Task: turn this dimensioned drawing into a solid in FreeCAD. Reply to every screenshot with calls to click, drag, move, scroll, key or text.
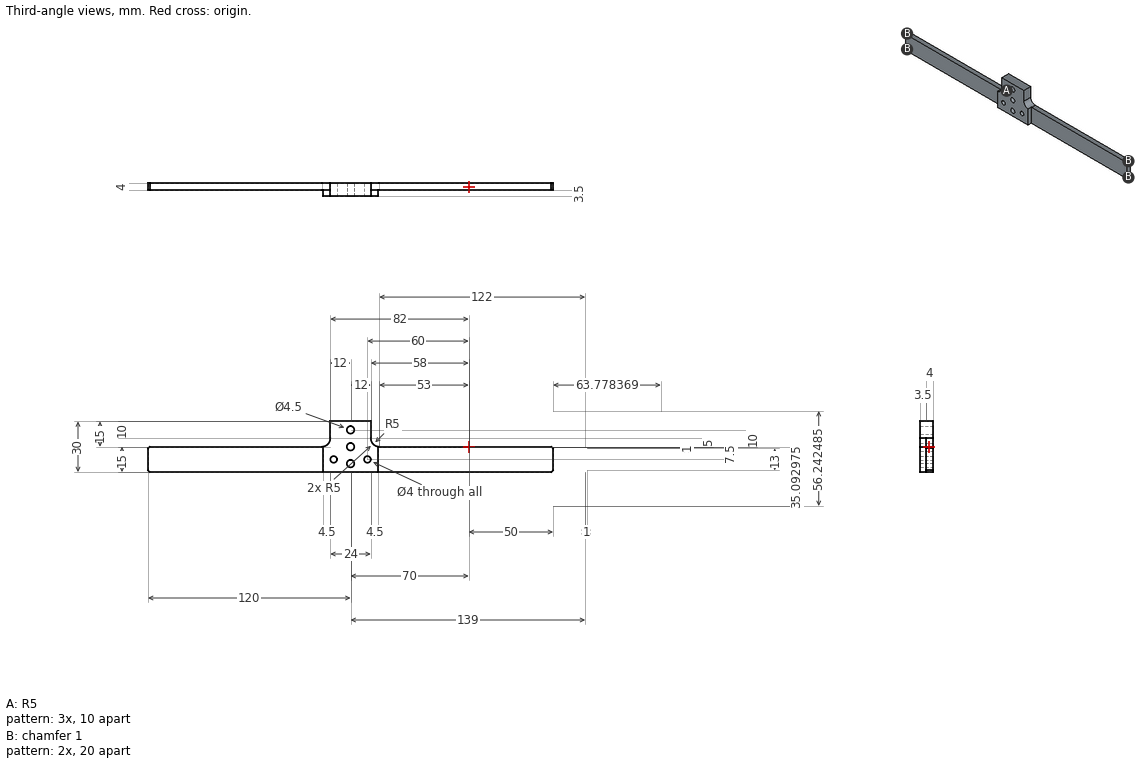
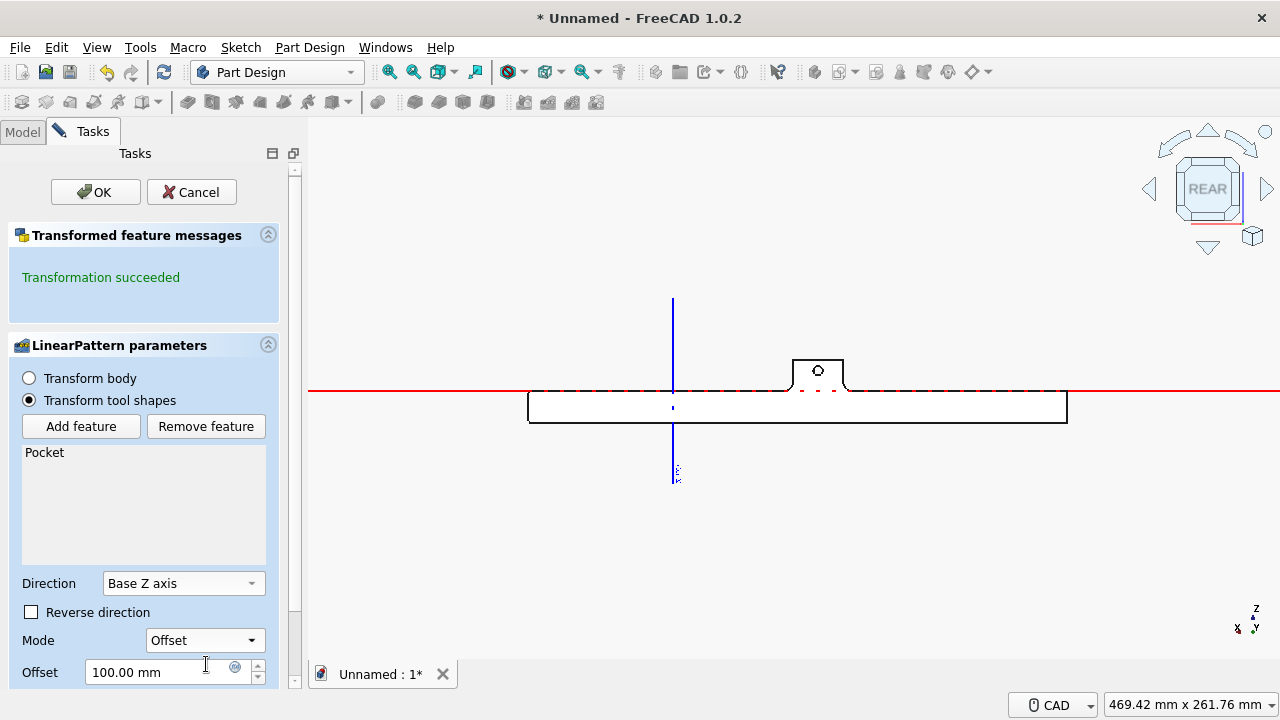
triple_click(168, 672)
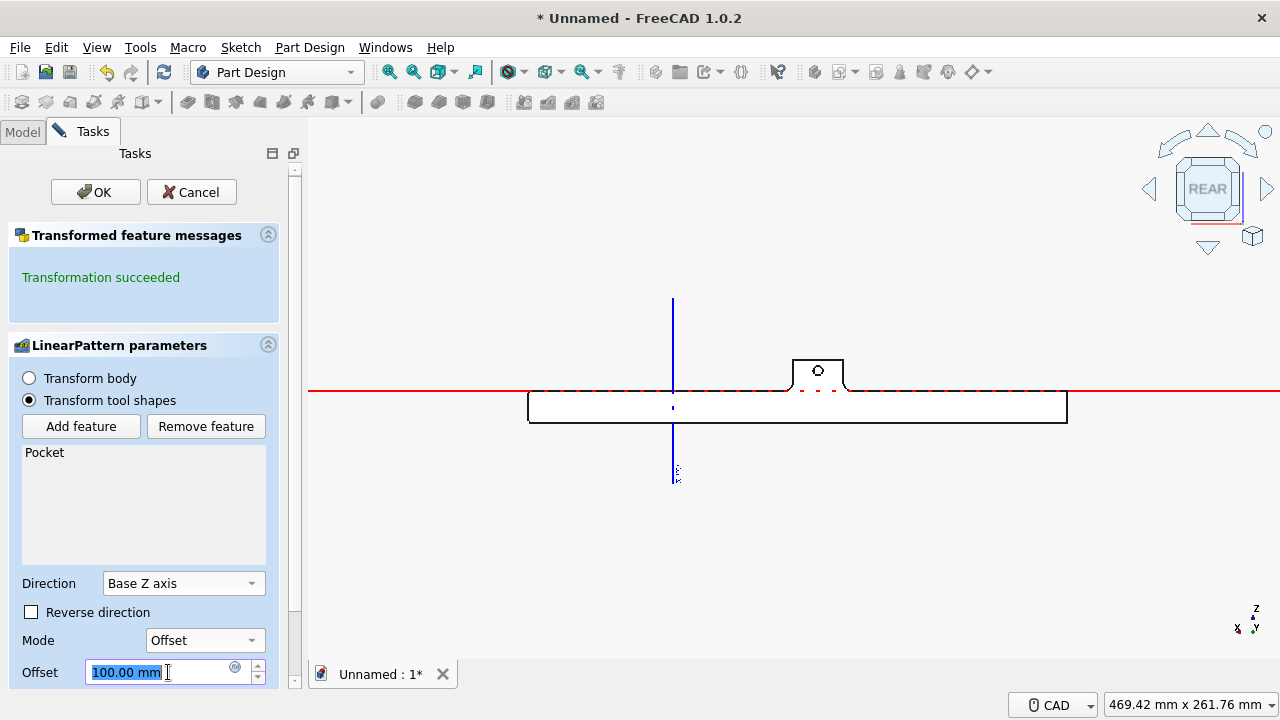
text(10)
key(Tab)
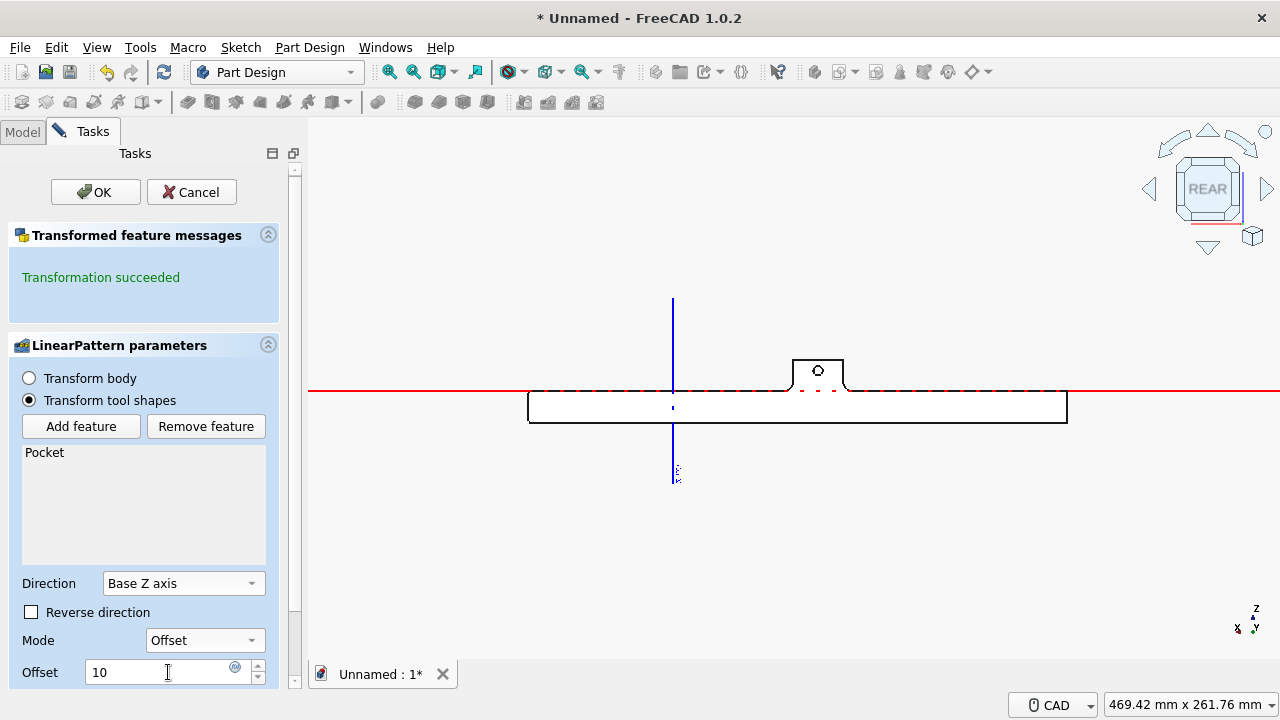
scroll(295, 426, down, 2)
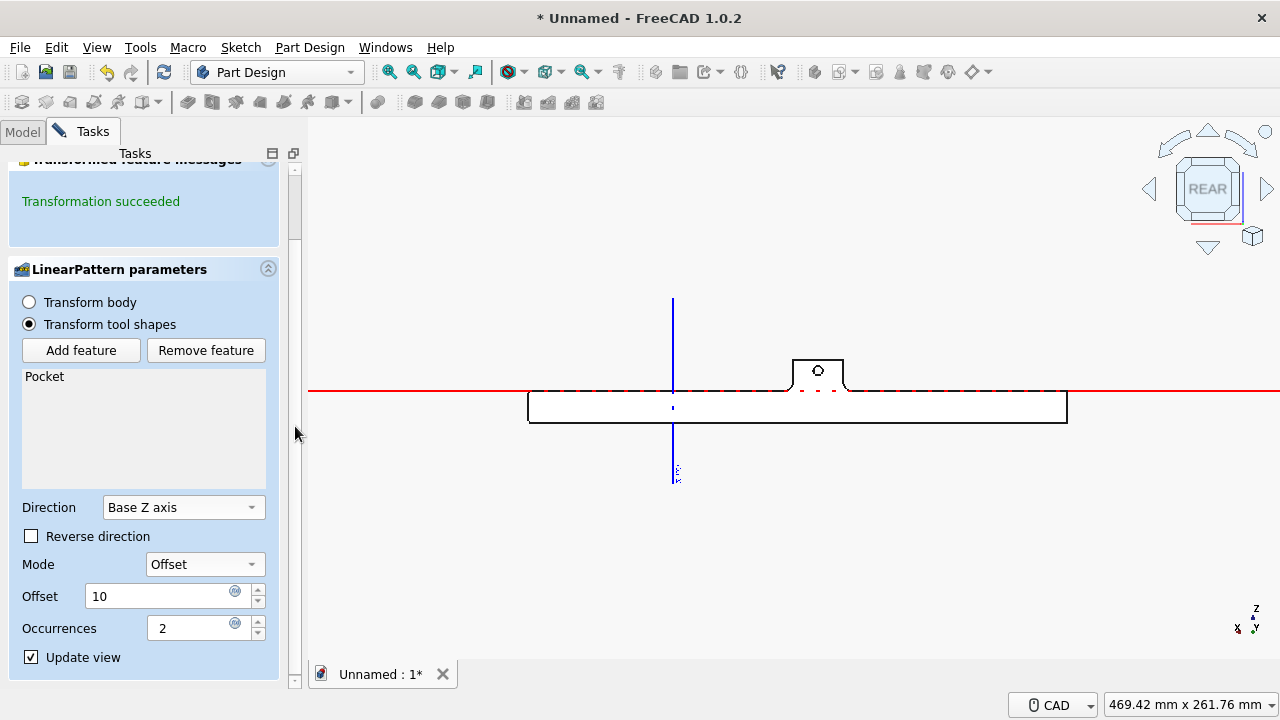
triple_click(198, 628)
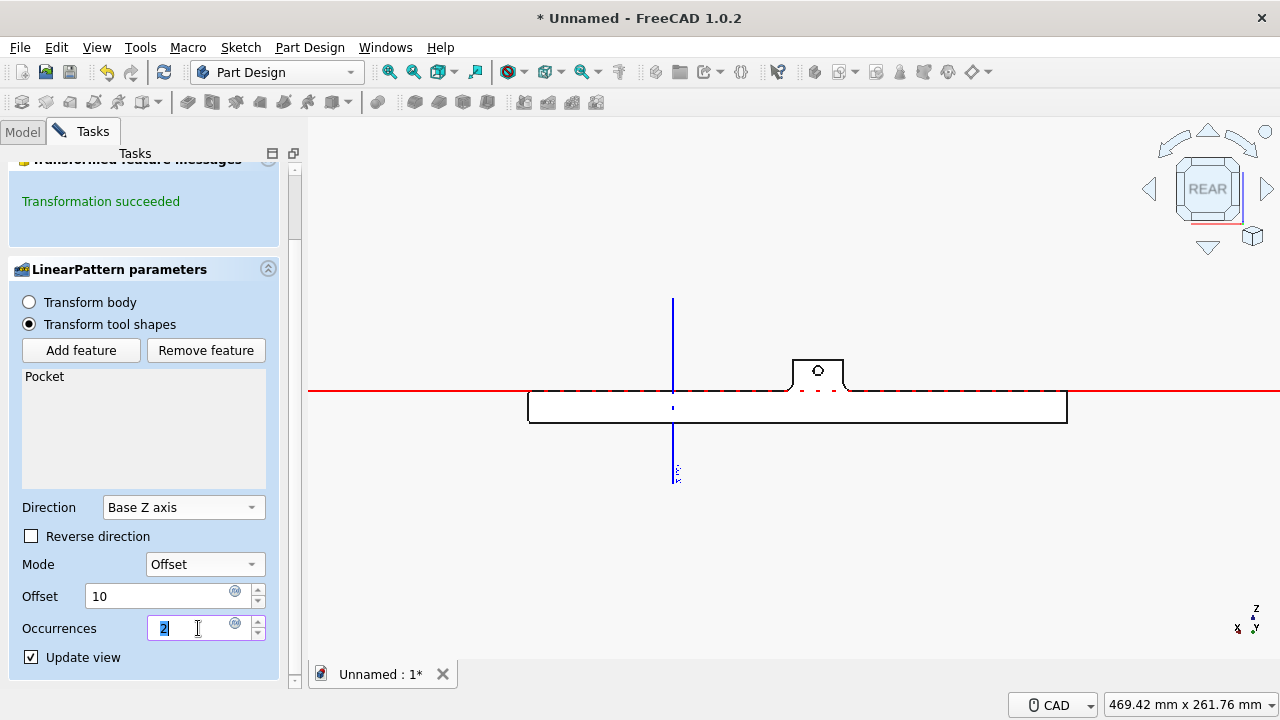
text(3)
key(Tab)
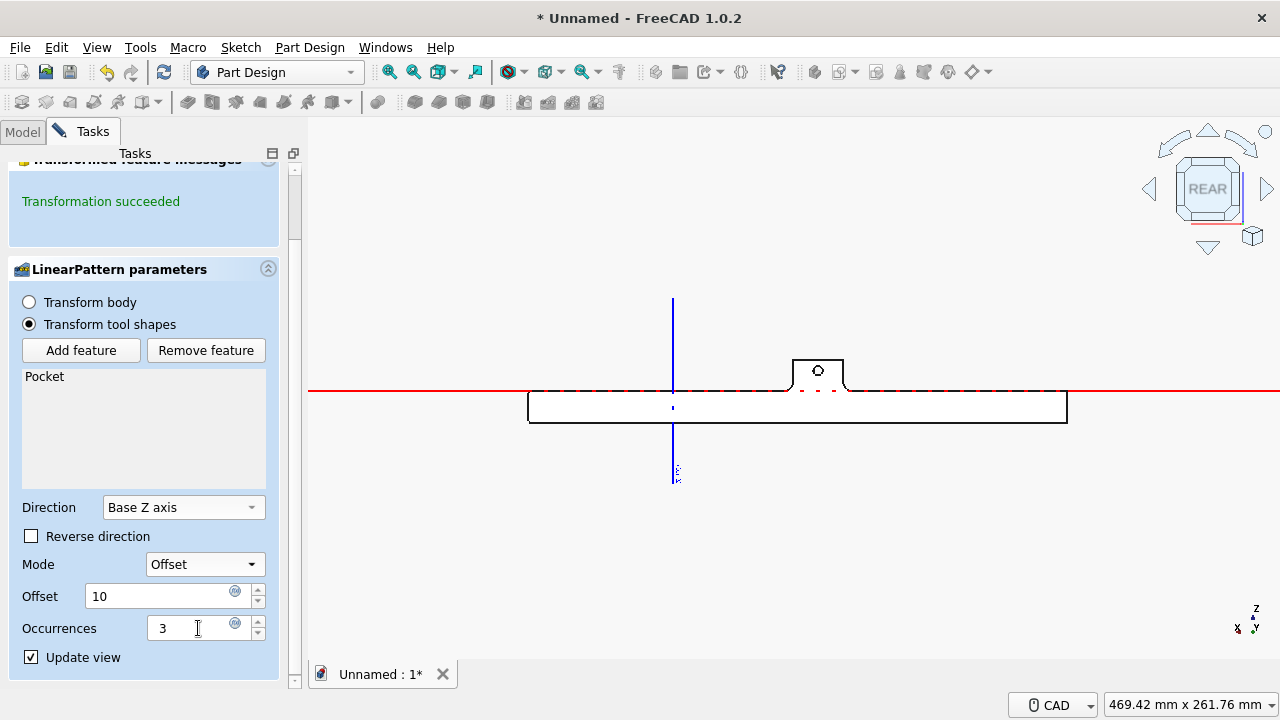
click(30, 536)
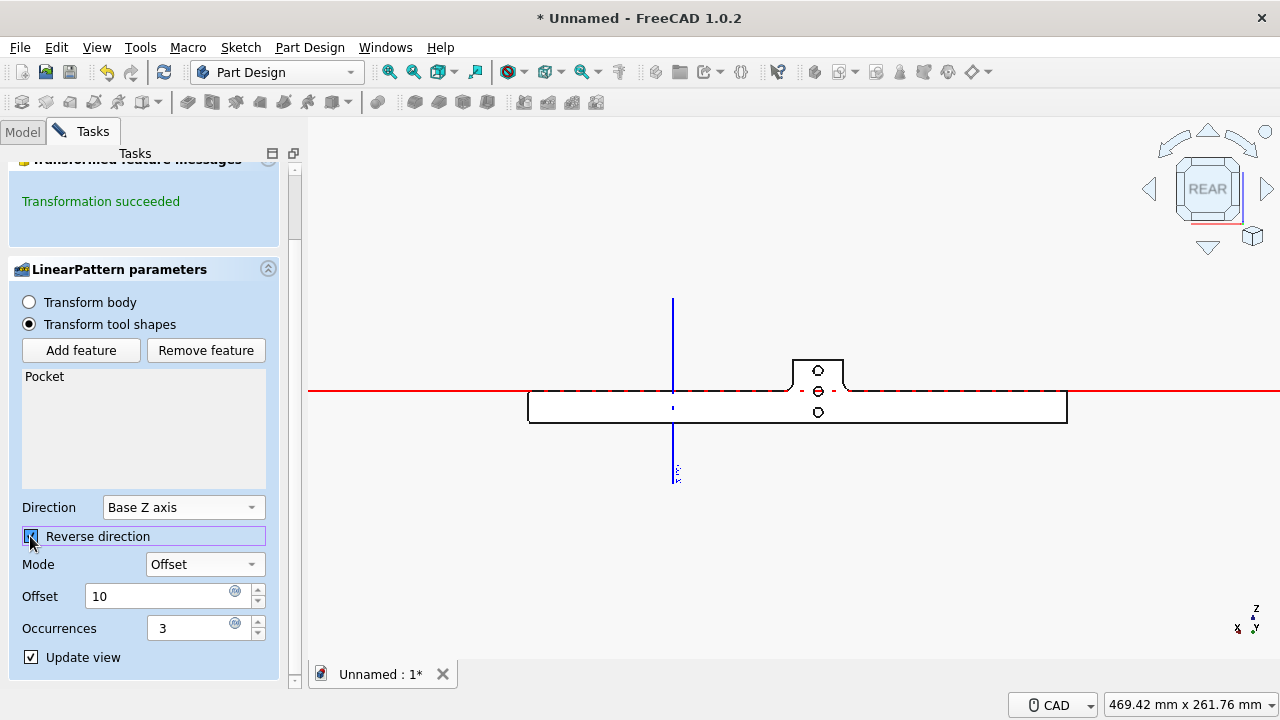
scroll(295, 426, up, 3)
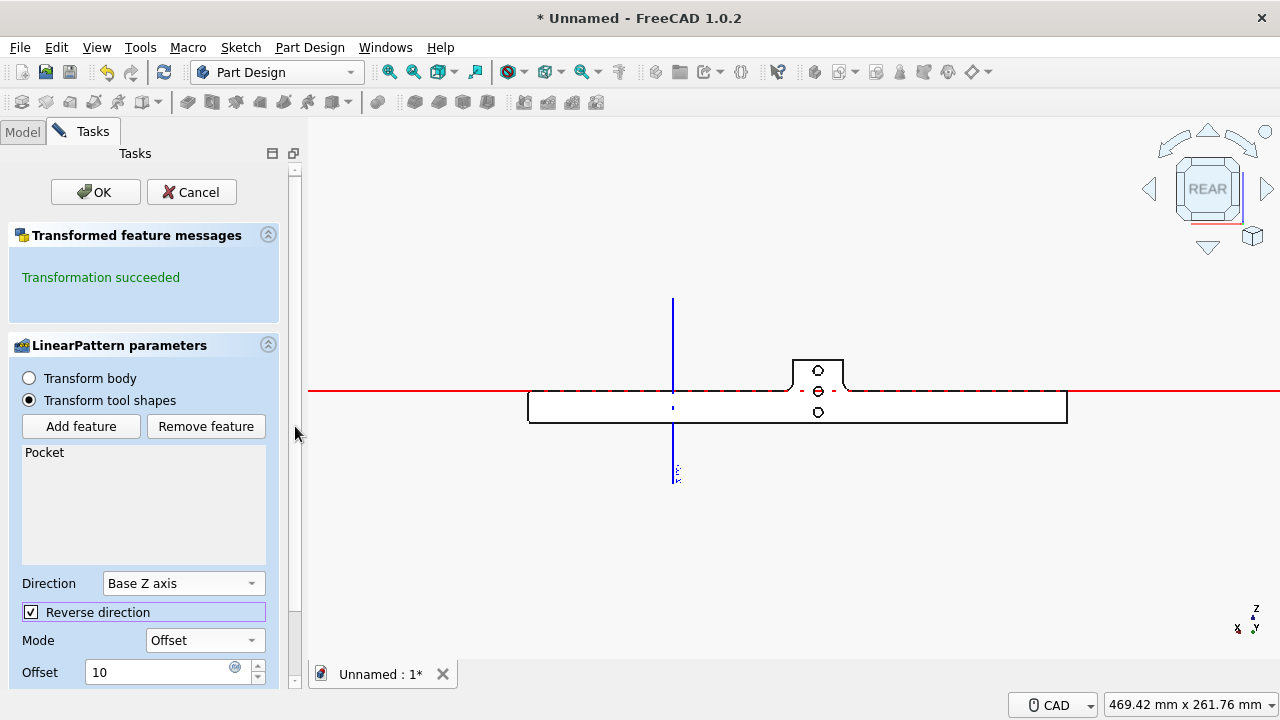
click(96, 192)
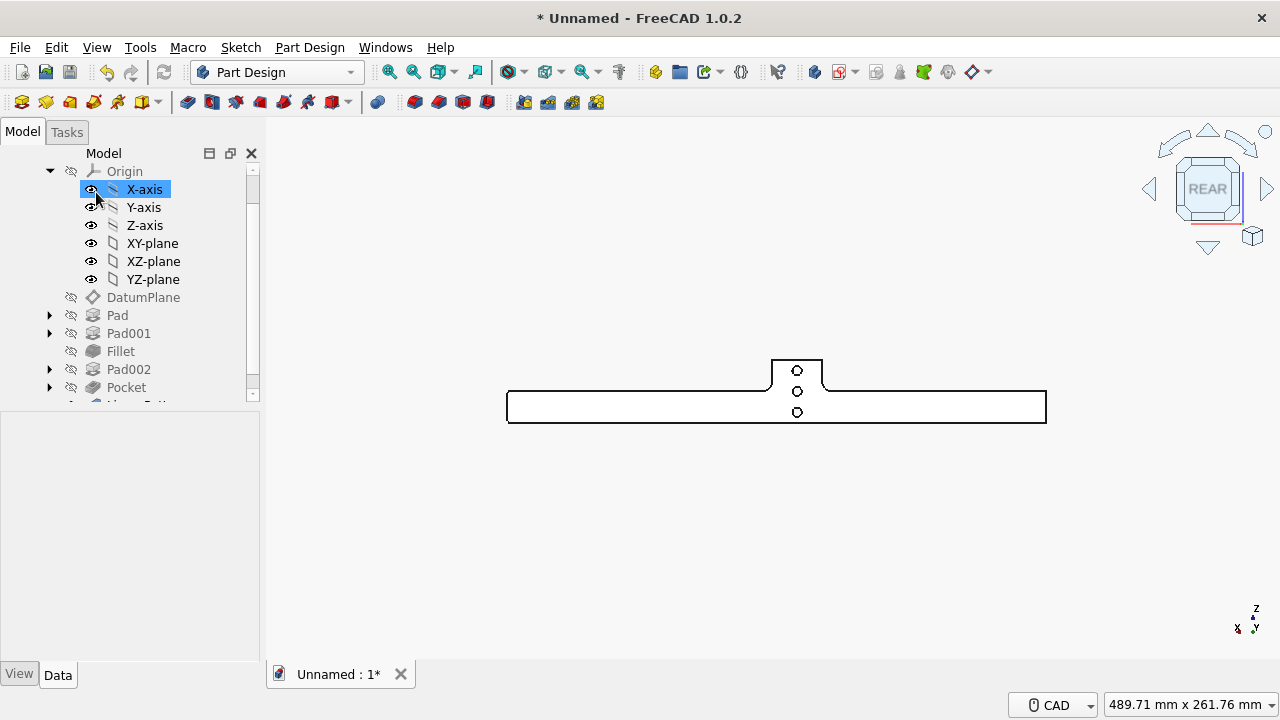
click(776, 399)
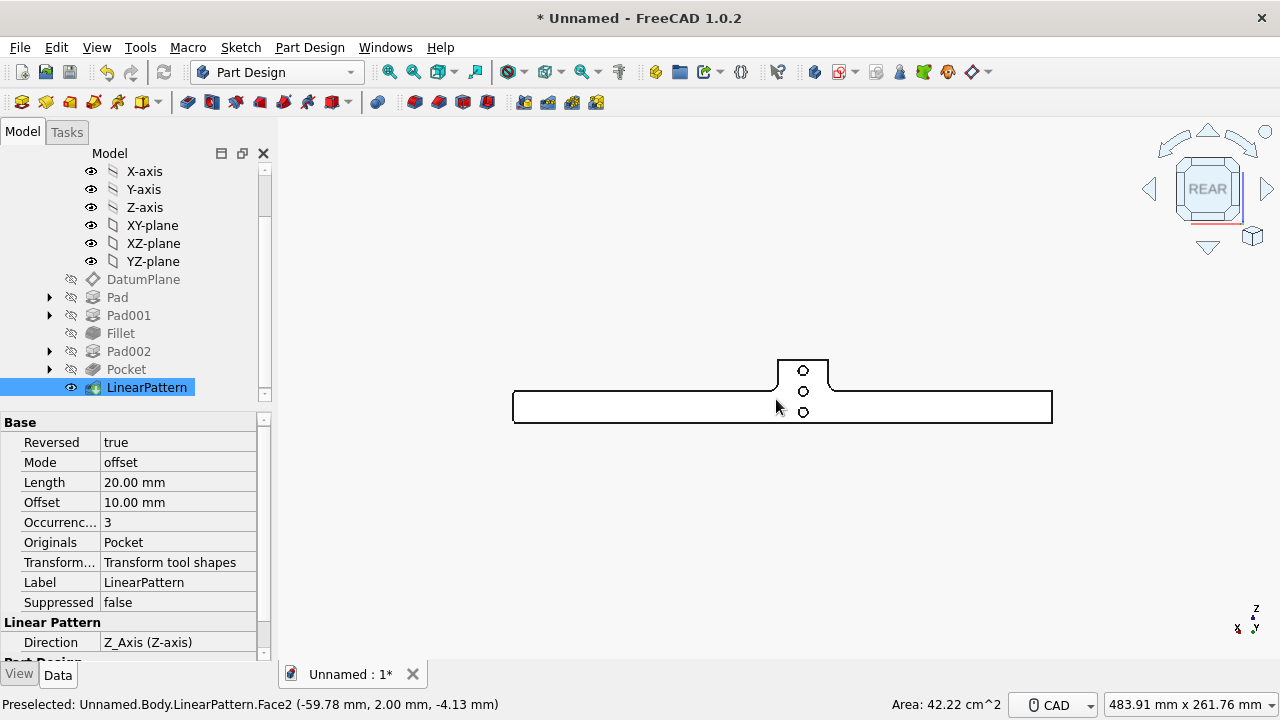
click(840, 72)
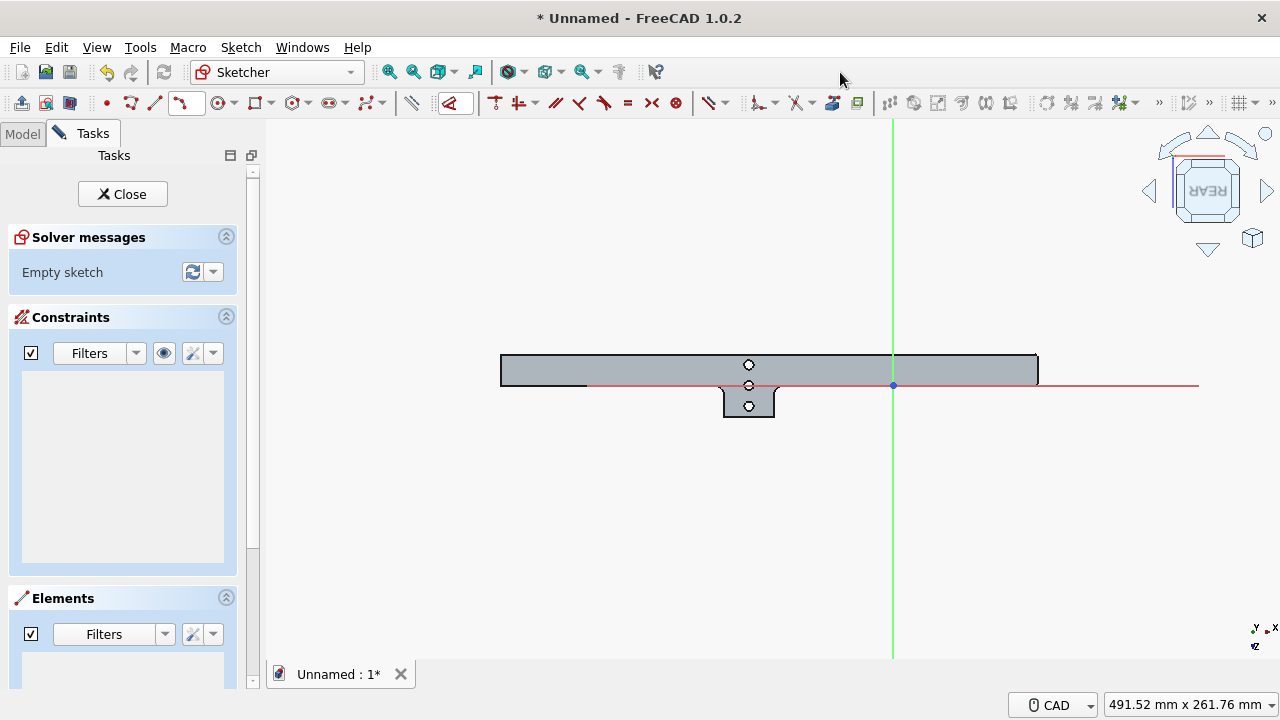
scroll(704, 389, down, 5)